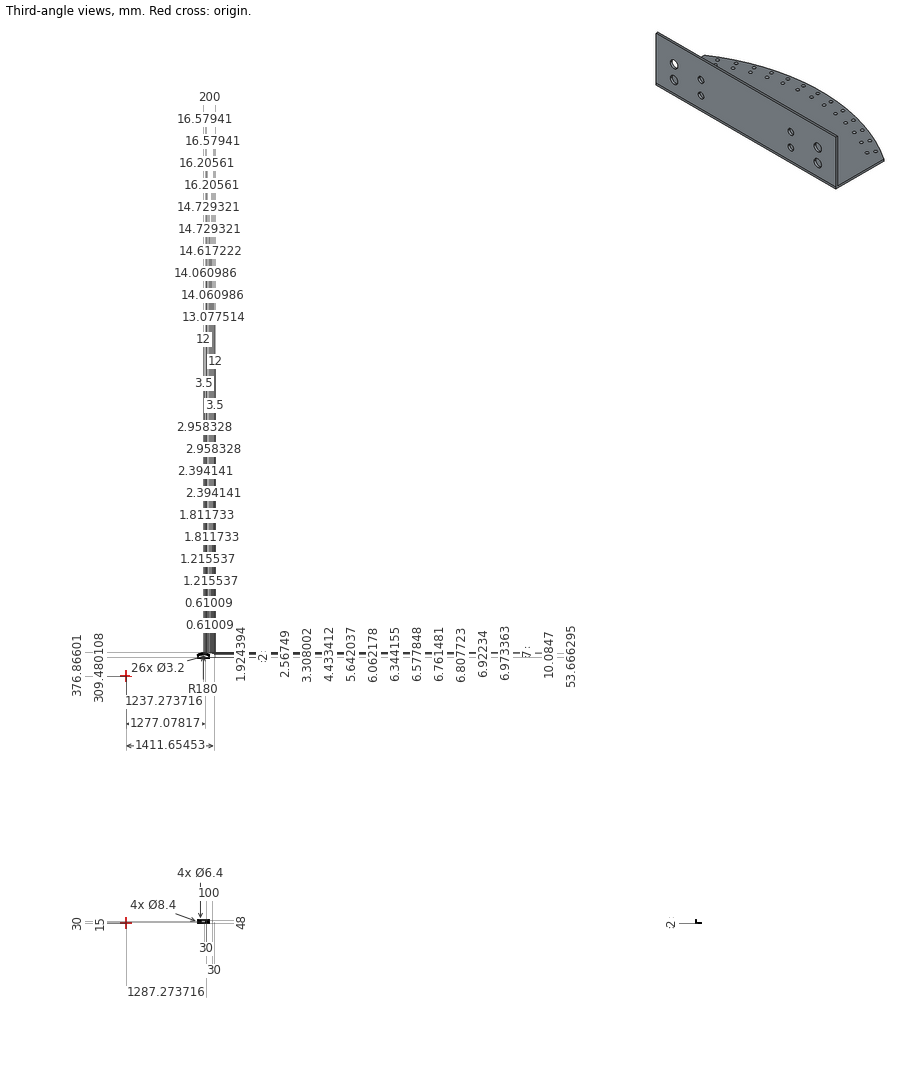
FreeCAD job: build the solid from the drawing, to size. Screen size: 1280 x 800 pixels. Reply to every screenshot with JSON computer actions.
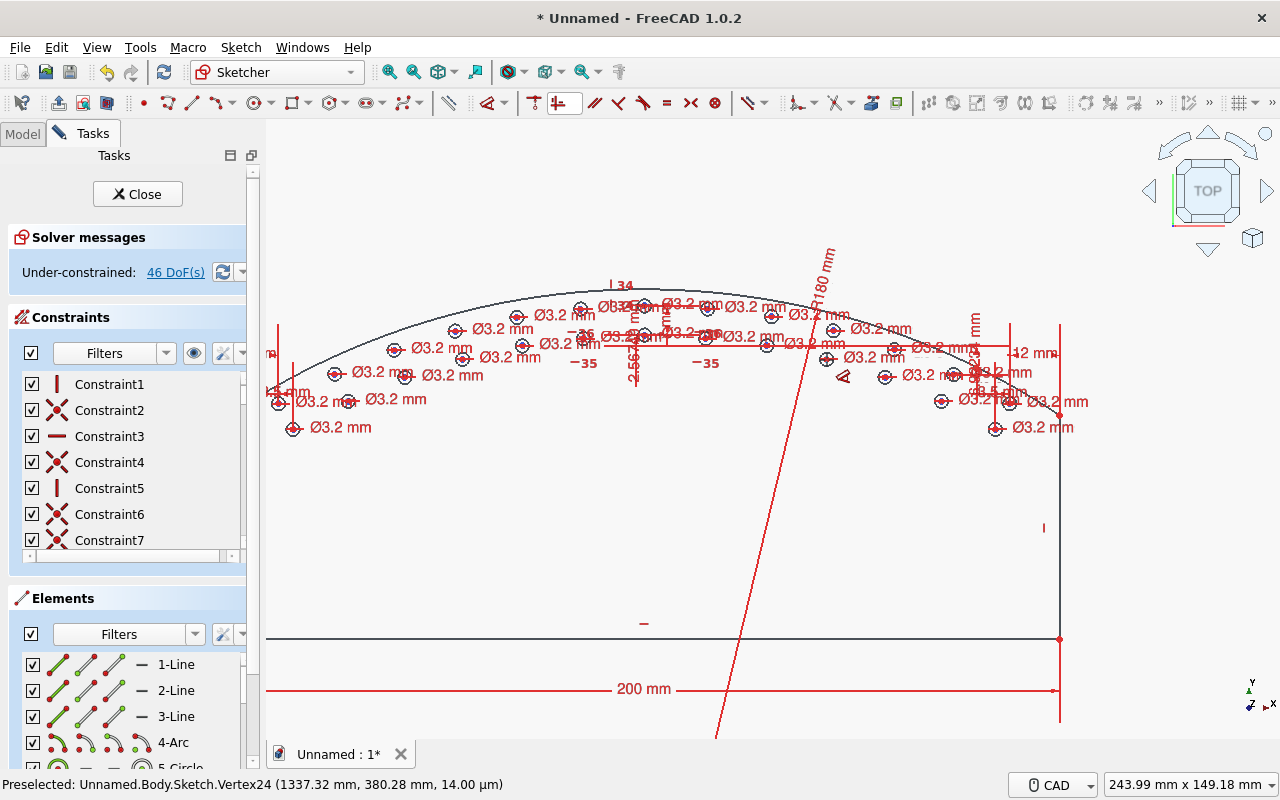
{"action": "left_click", "coordinate": [827, 359]}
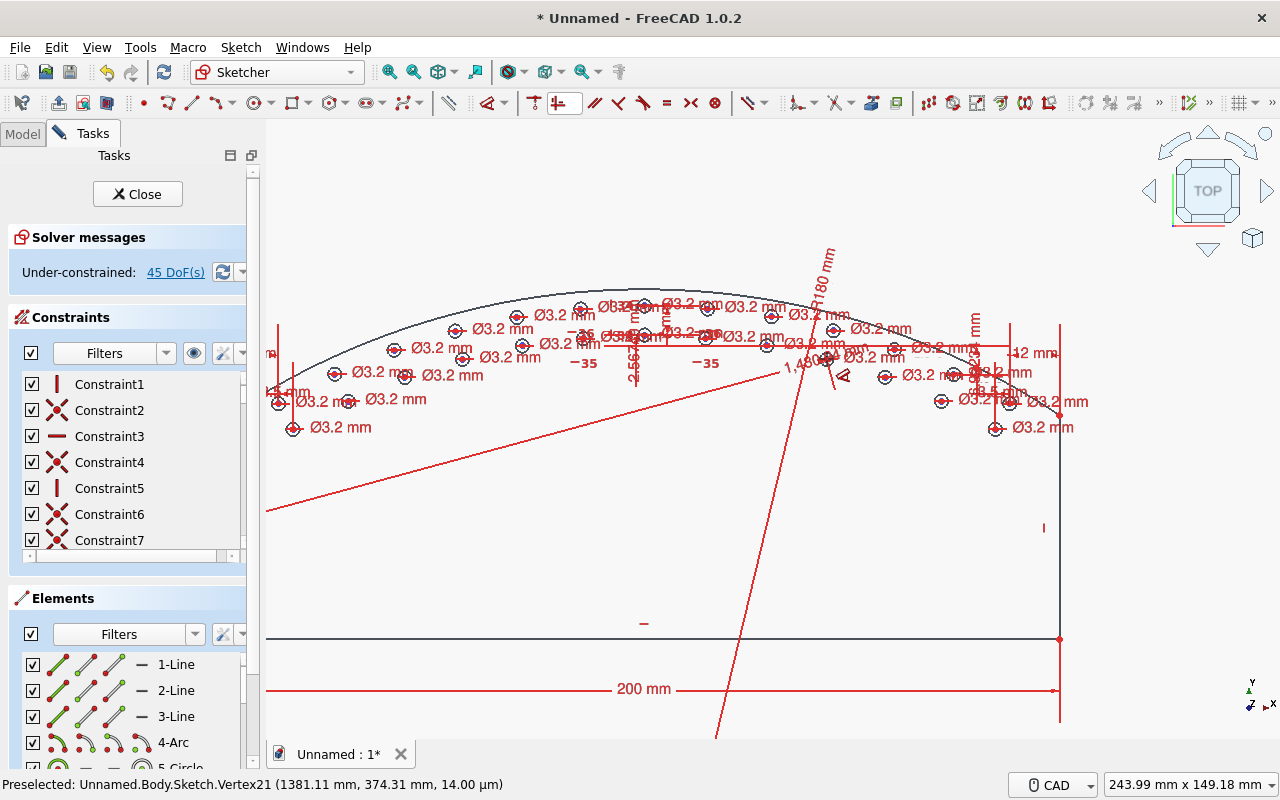
{"action": "left_click", "coordinate": [772, 317]}
{"action": "left_click", "coordinate": [861, 338]}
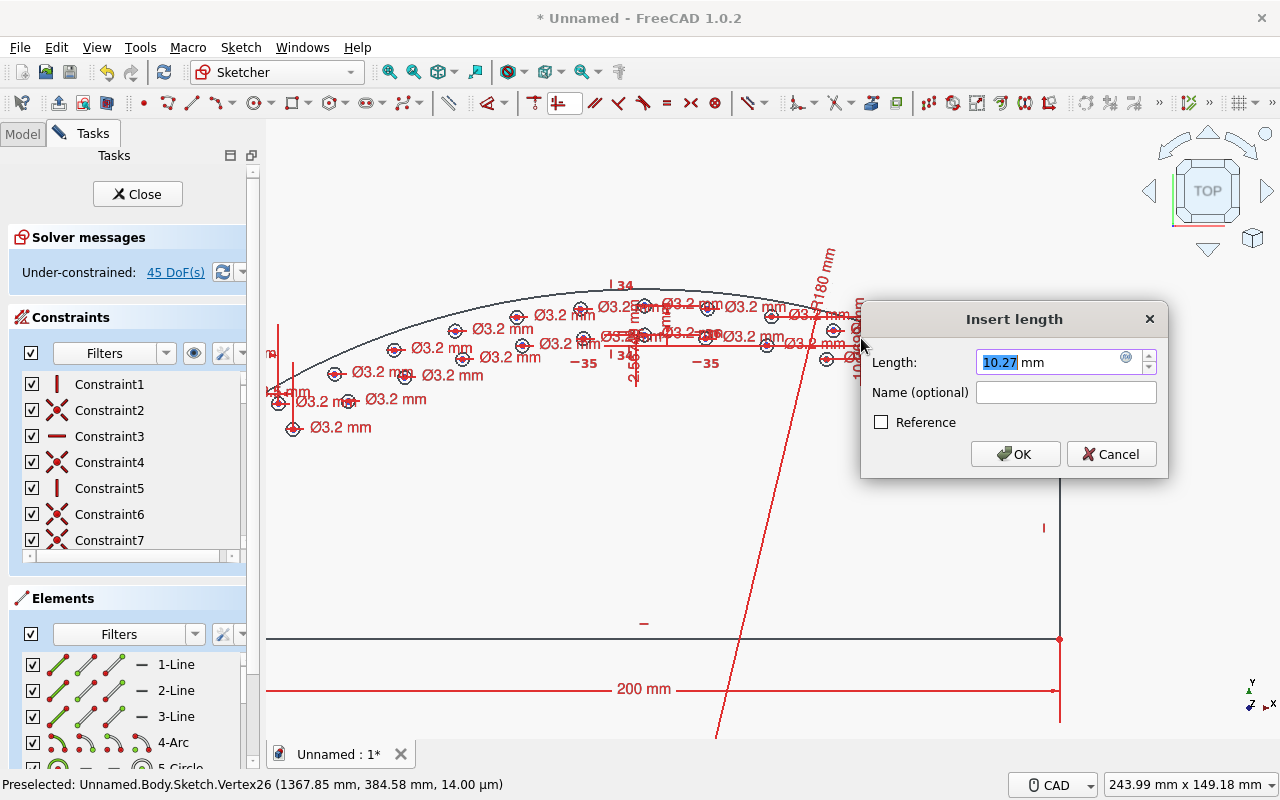
{"action": "type", "text": "10.0847"}
{"action": "key", "text": "Return"}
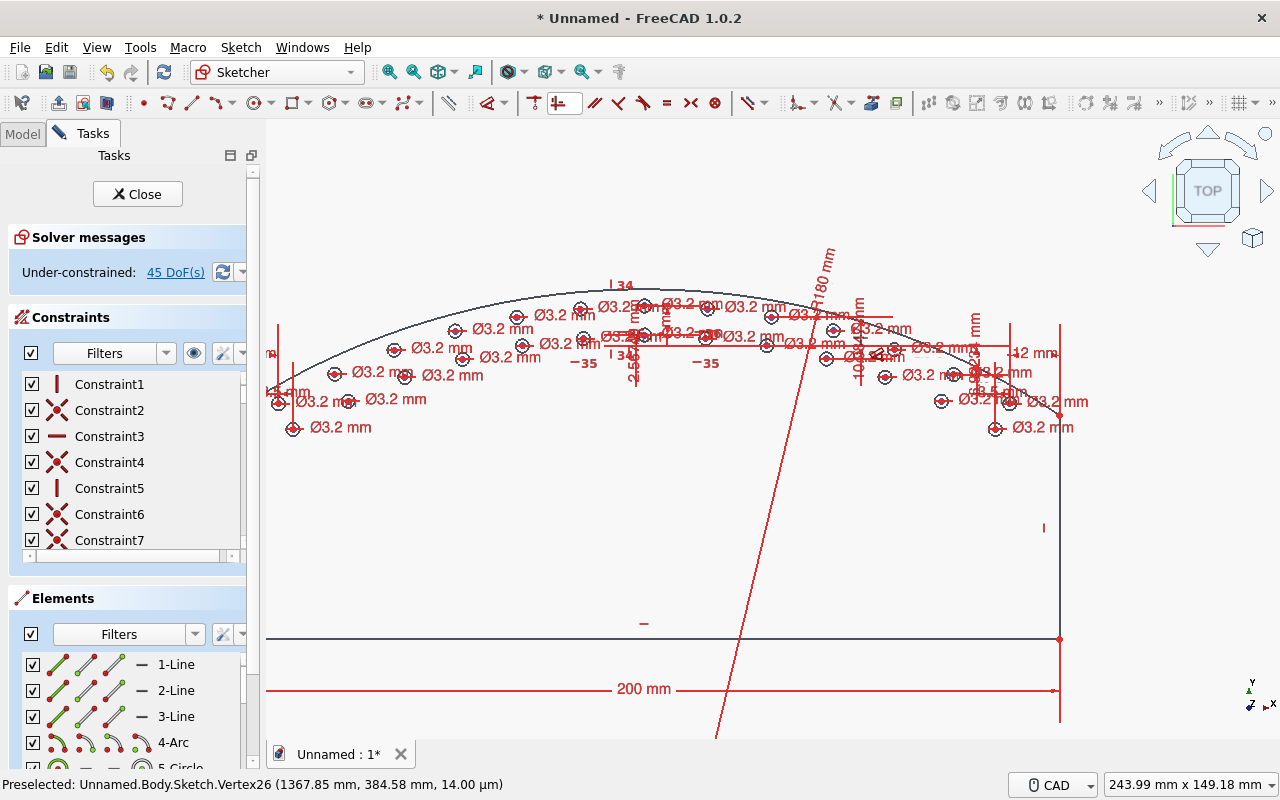
{"action": "scroll", "coordinate": [706, 339], "scroll_direction": "up", "scroll_amount": 14}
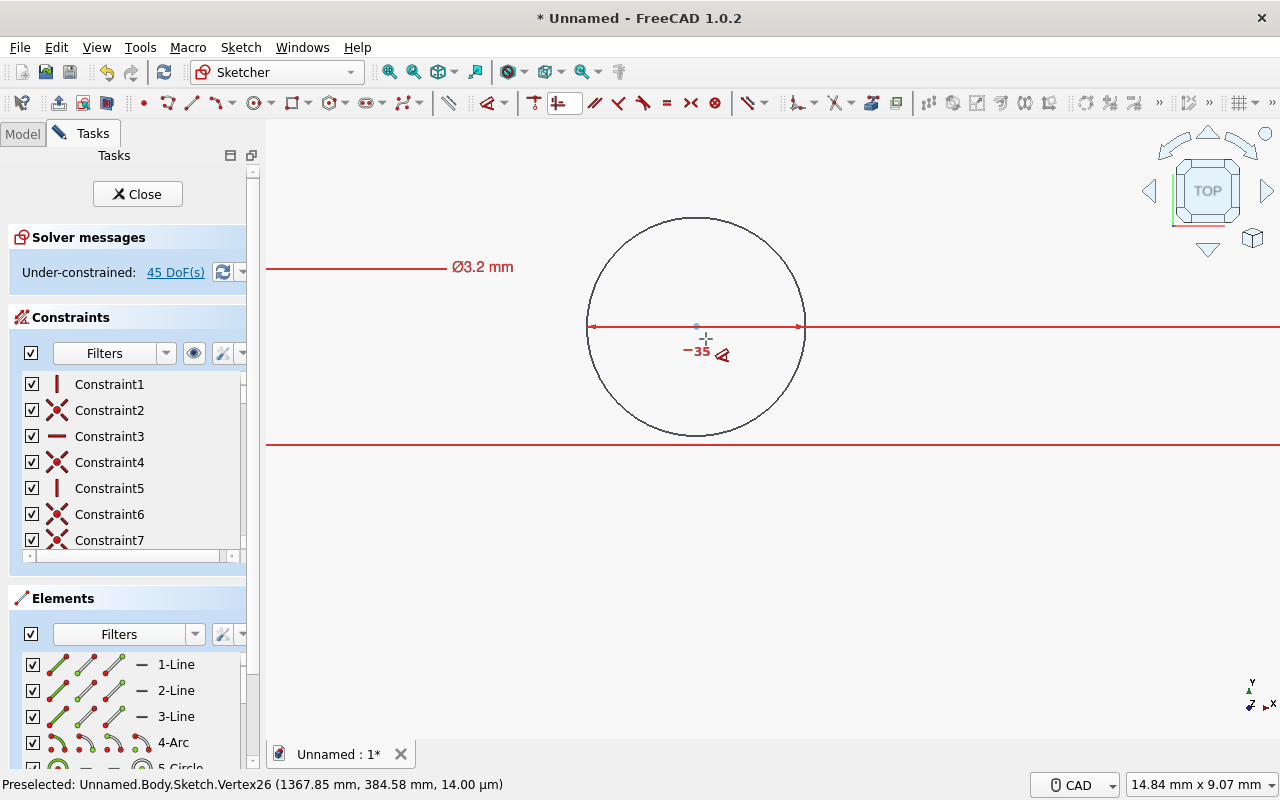
{"action": "left_click", "coordinate": [696, 327]}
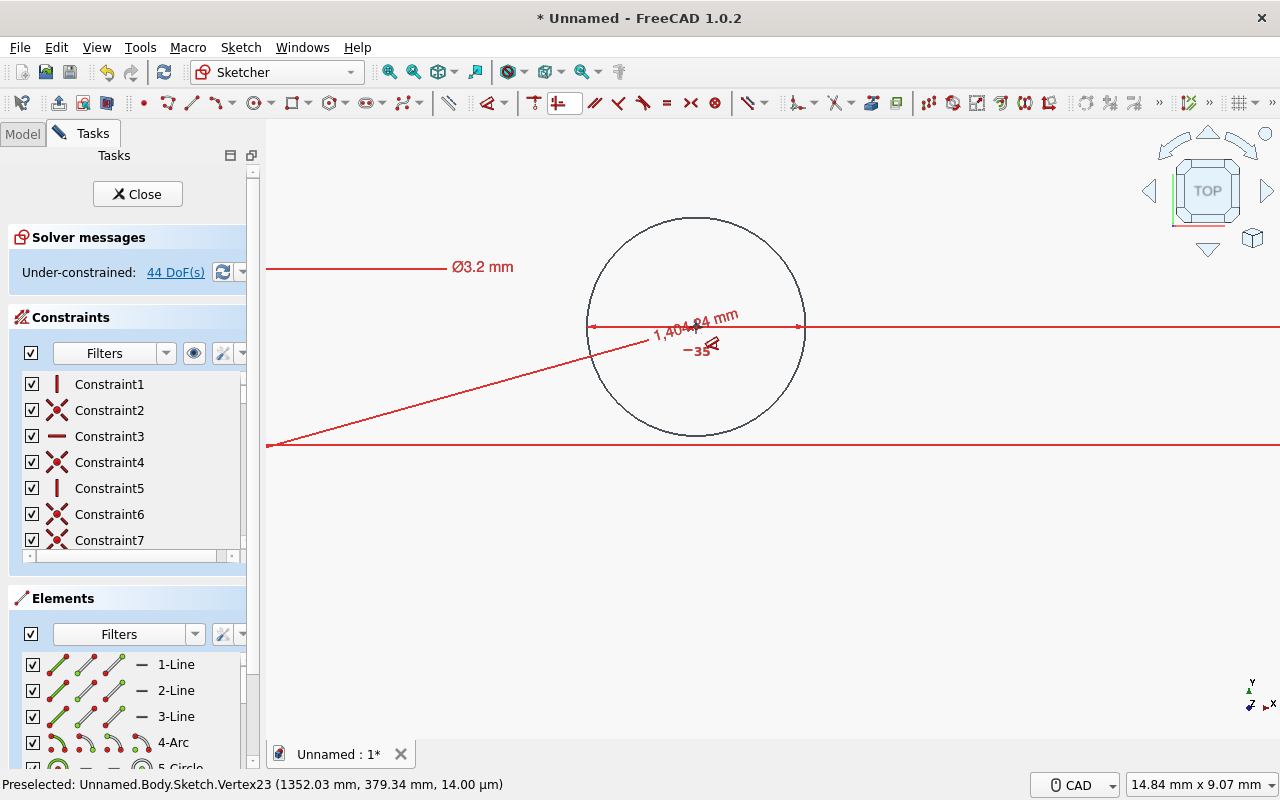
{"action": "scroll", "coordinate": [758, 327], "scroll_direction": "down", "scroll_amount": 15}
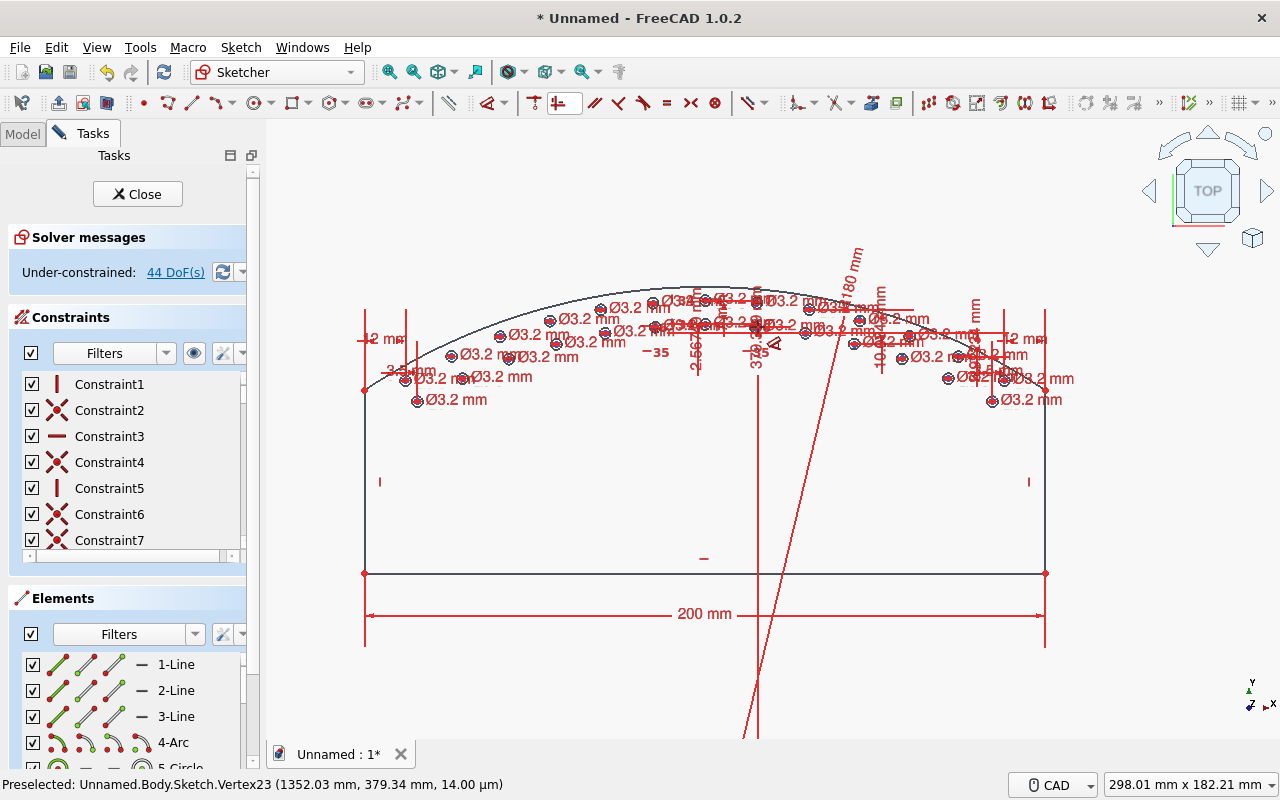
{"action": "scroll", "coordinate": [757, 303], "scroll_direction": "up", "scroll_amount": 15}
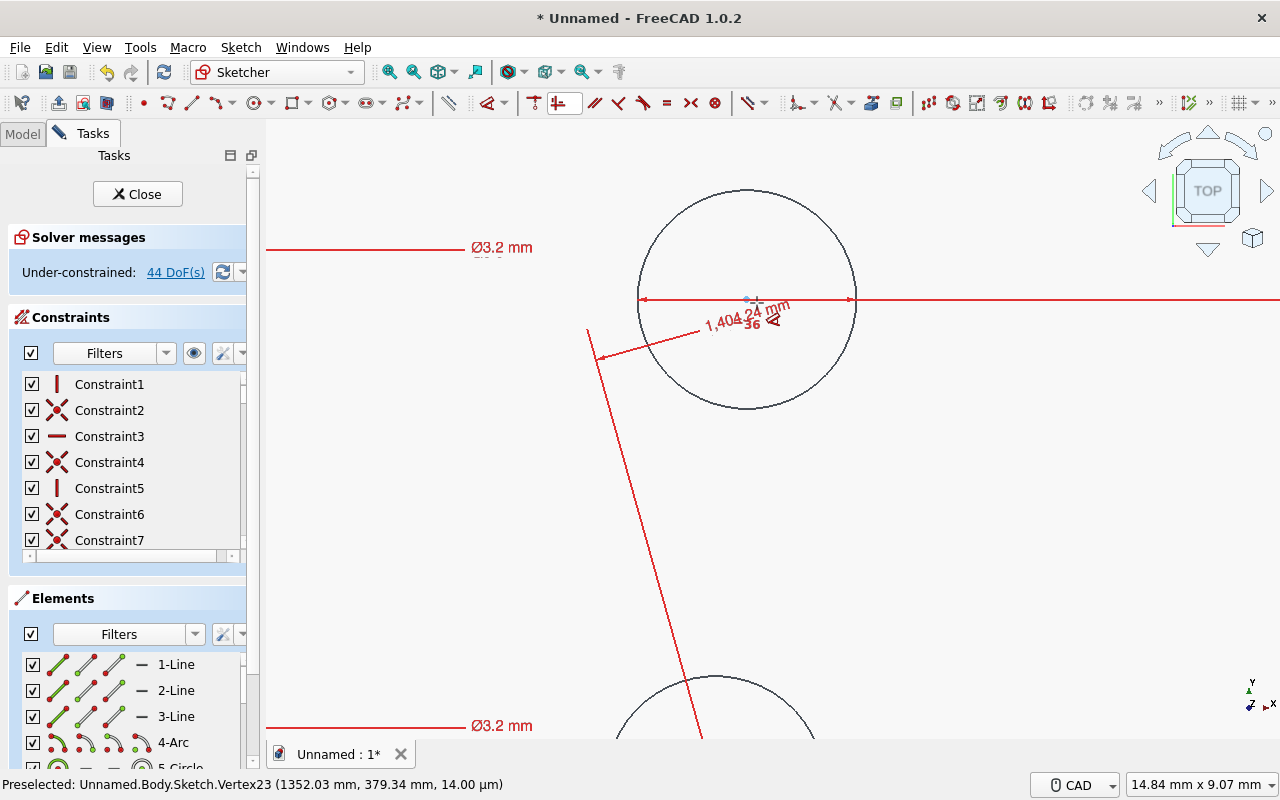
{"action": "left_click", "coordinate": [747, 300]}
{"action": "left_click", "coordinate": [731, 266]}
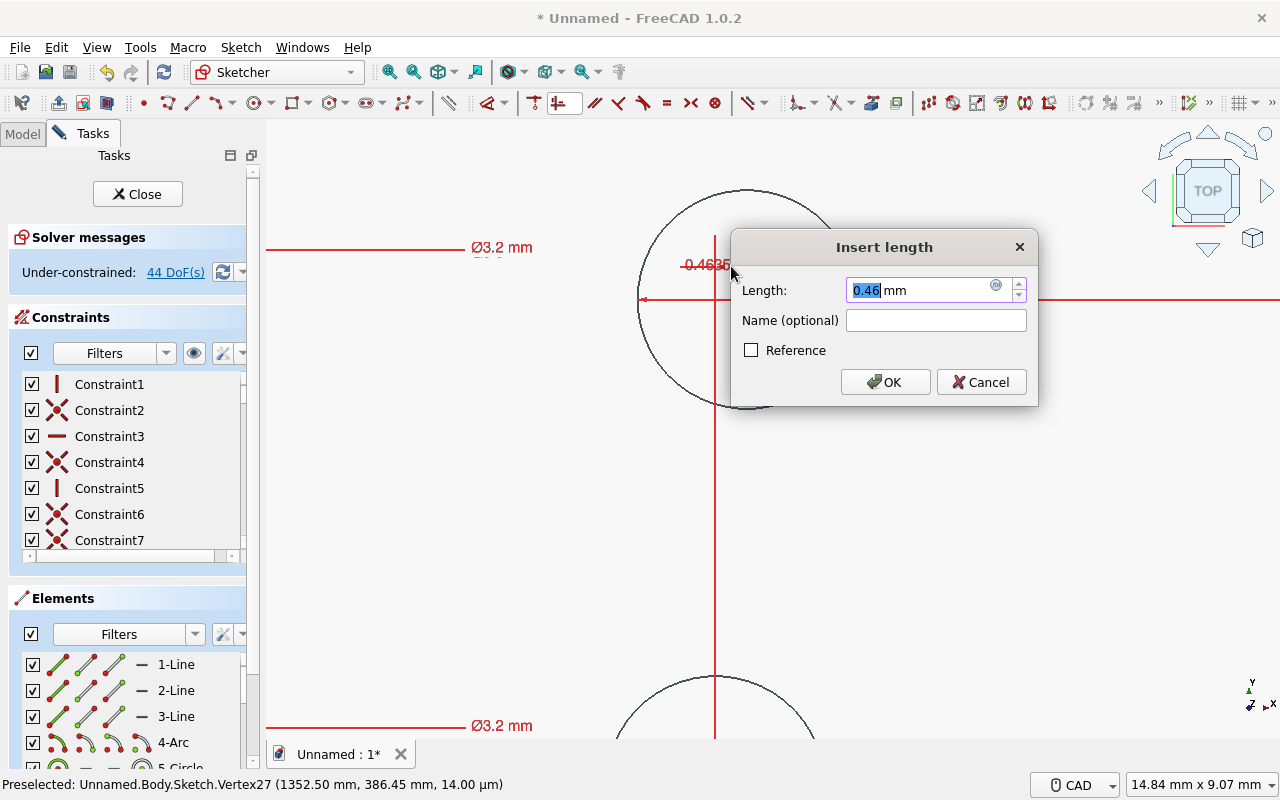
{"action": "type", "text": "0.61009"}
{"action": "key", "text": "Return"}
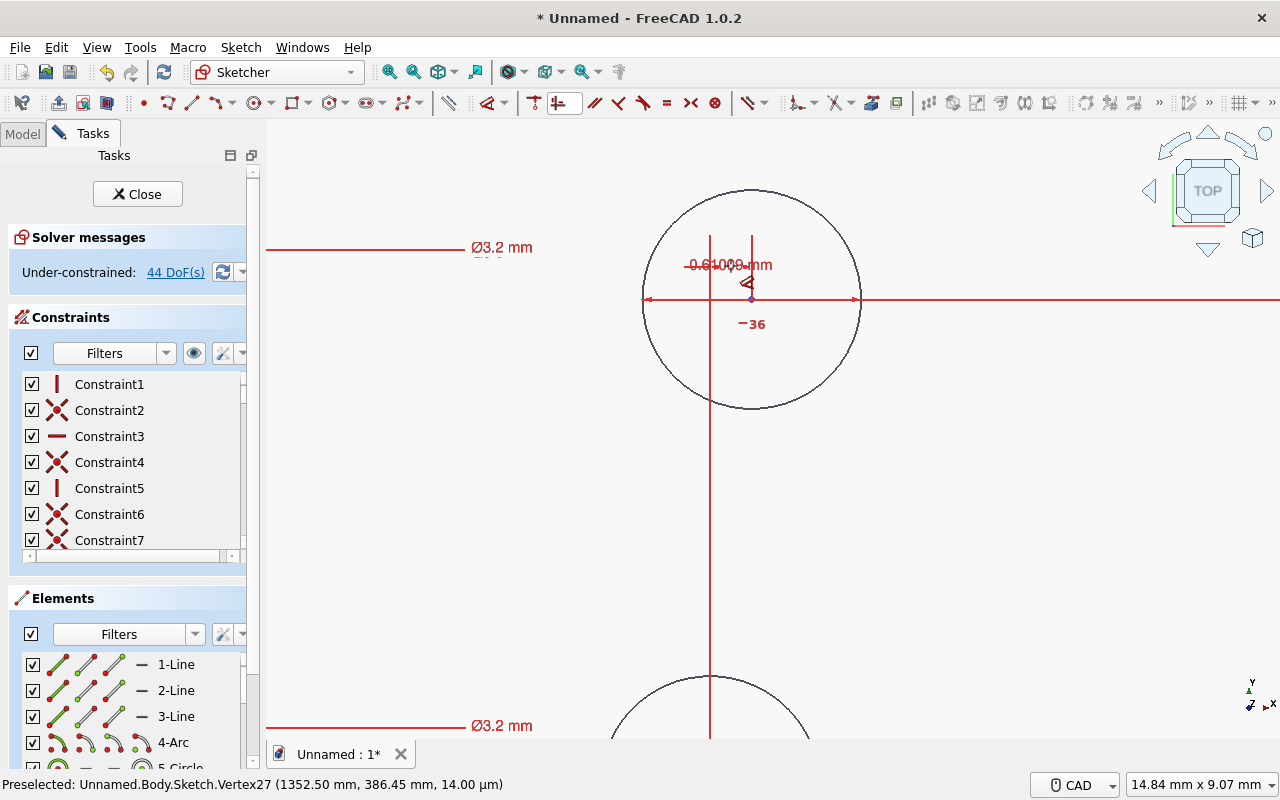
{"action": "scroll", "coordinate": [757, 303], "scroll_direction": "down", "scroll_amount": 15}